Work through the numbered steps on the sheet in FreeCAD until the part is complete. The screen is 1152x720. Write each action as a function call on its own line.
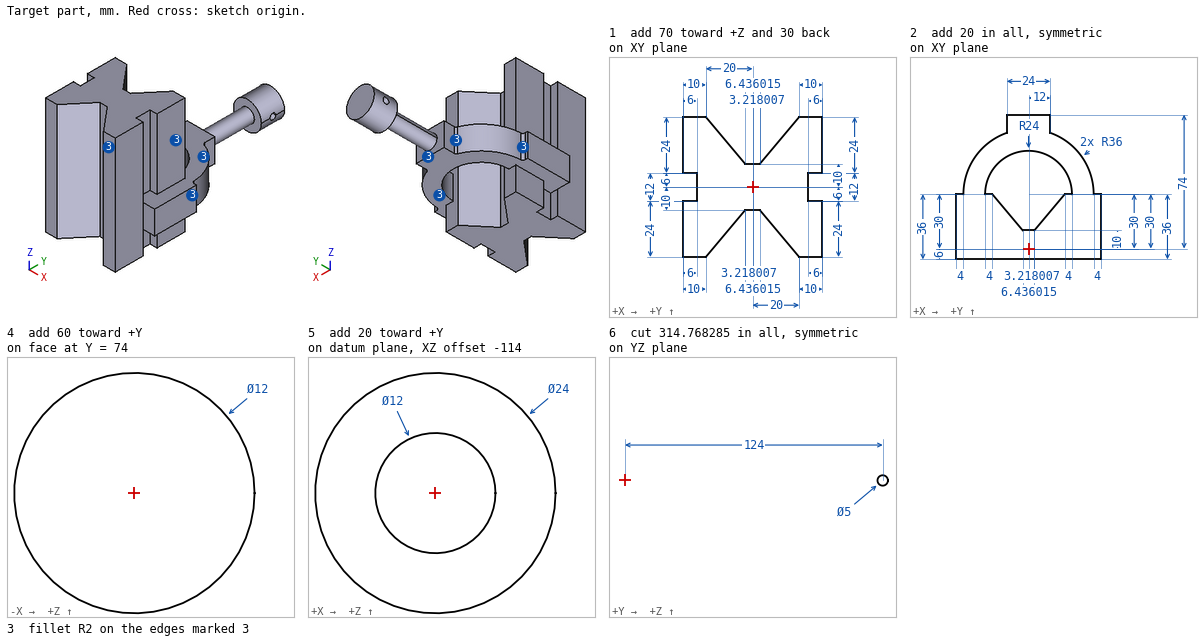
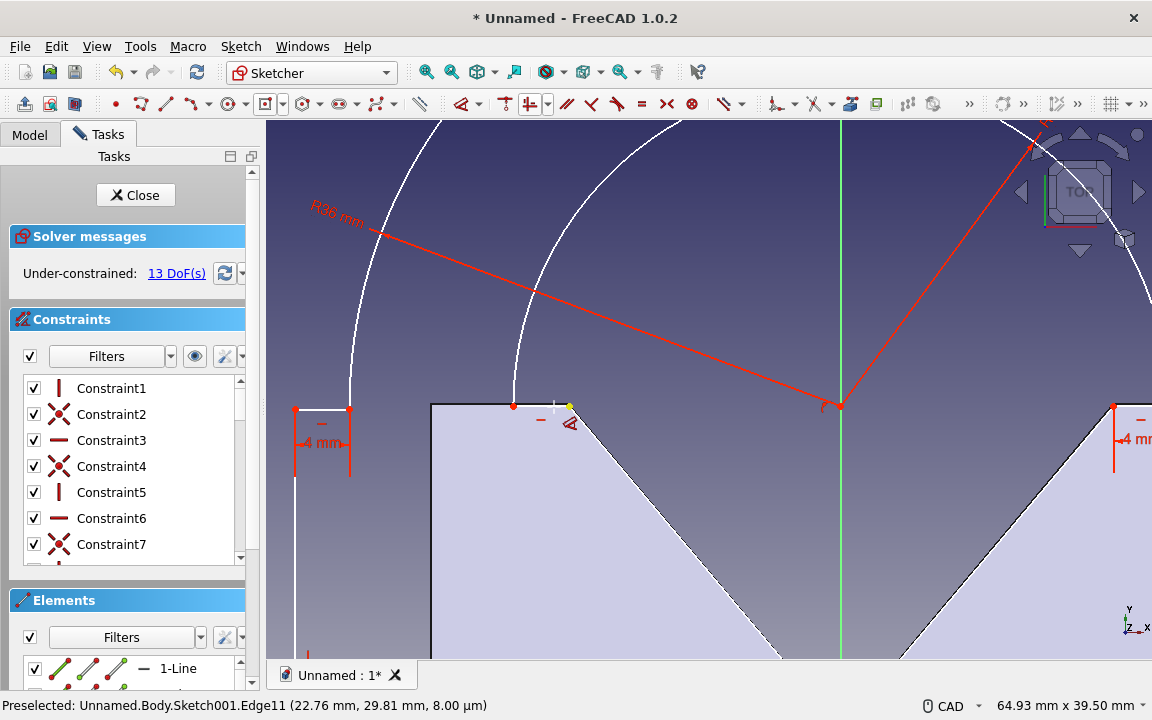
click(552, 406)
click(541, 440)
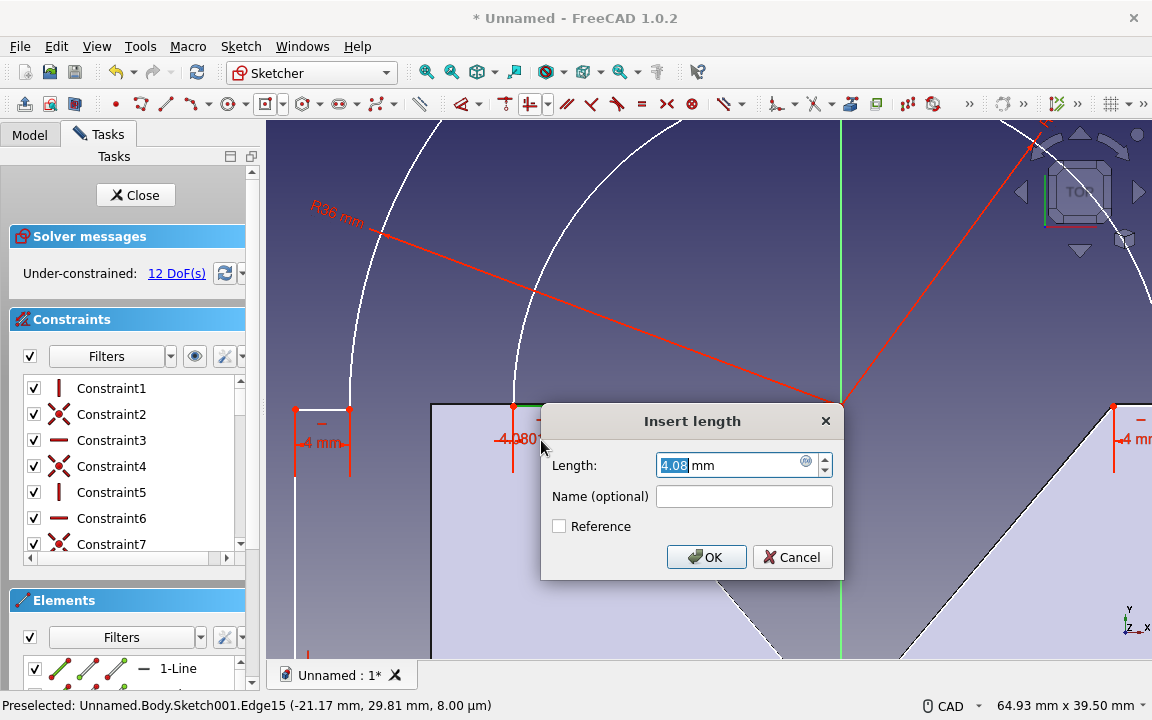
text(4)
key(Return)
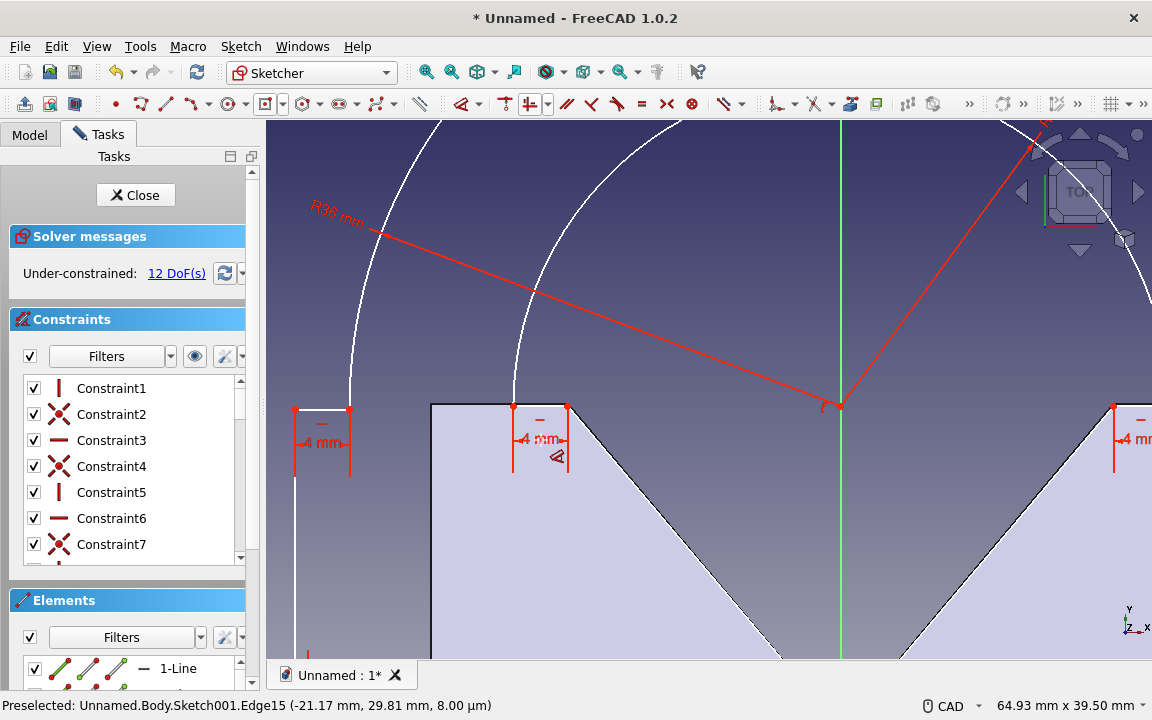
scroll(554, 407, down, 6)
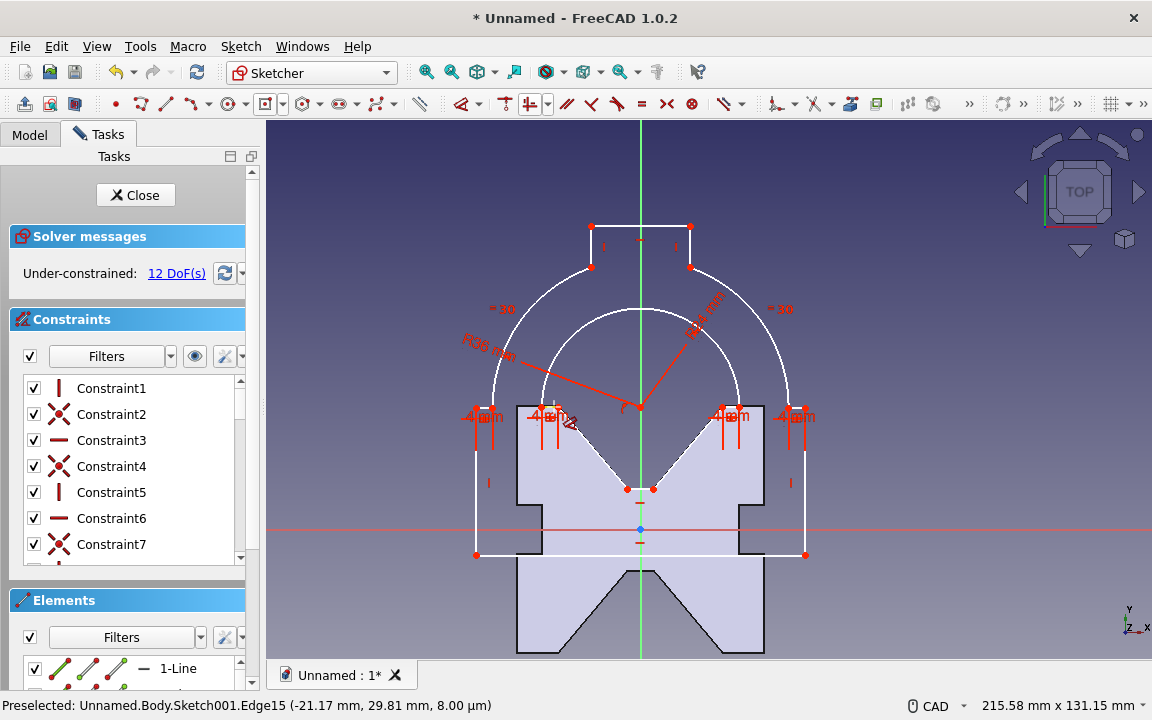
click(660, 226)
click(618, 192)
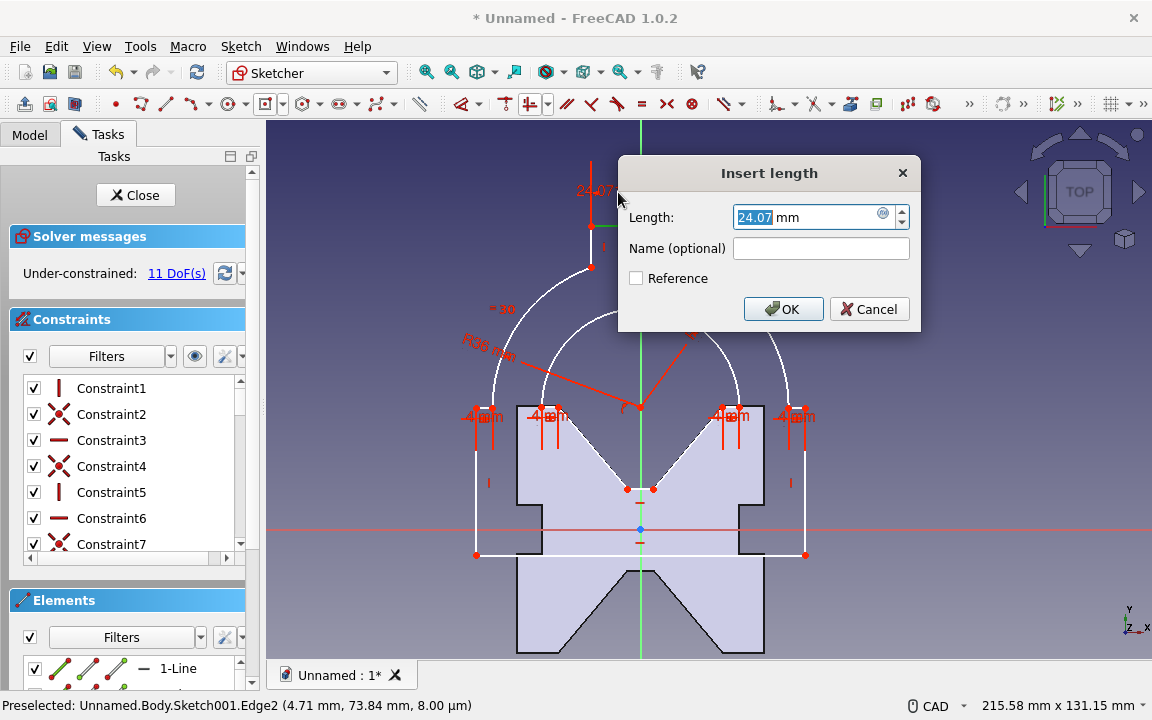
text(24)
key(Return)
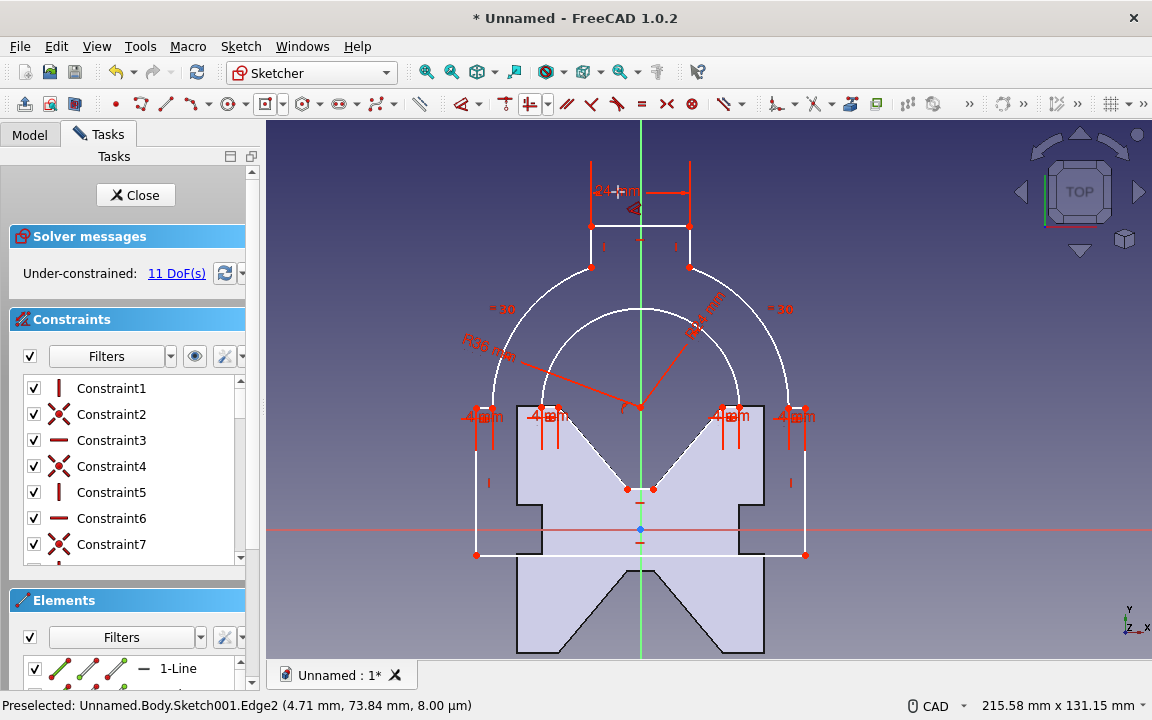
click(476, 453)
click(442, 482)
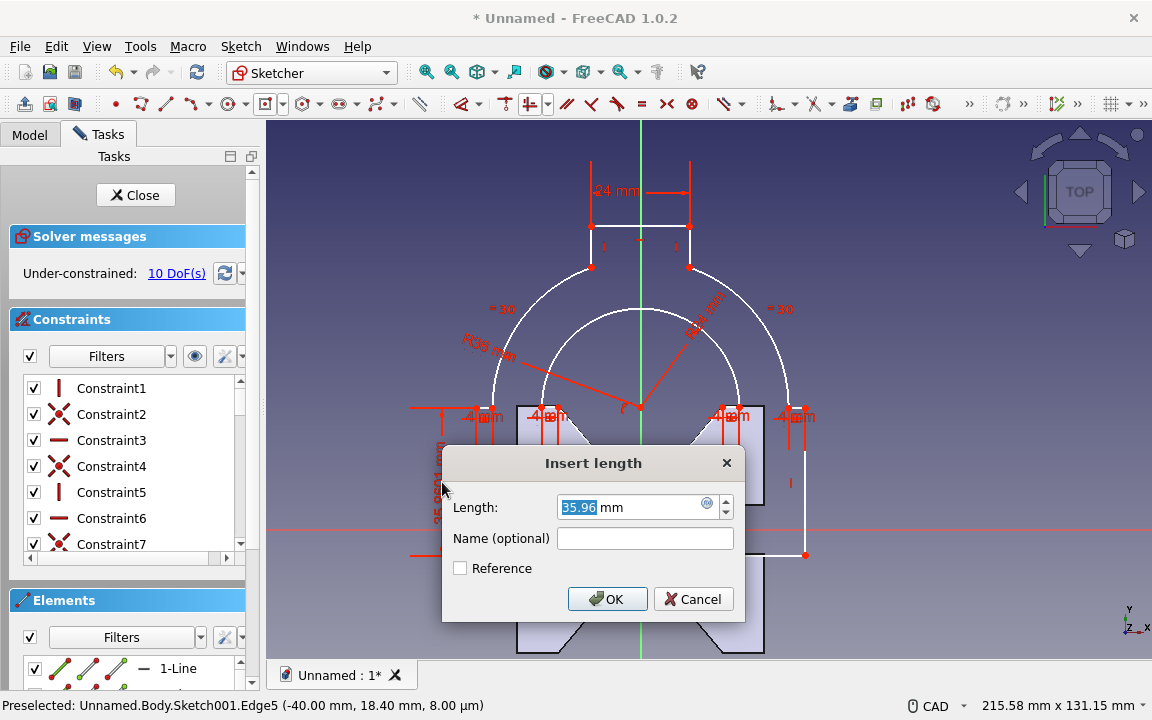
text(36)
key(Return)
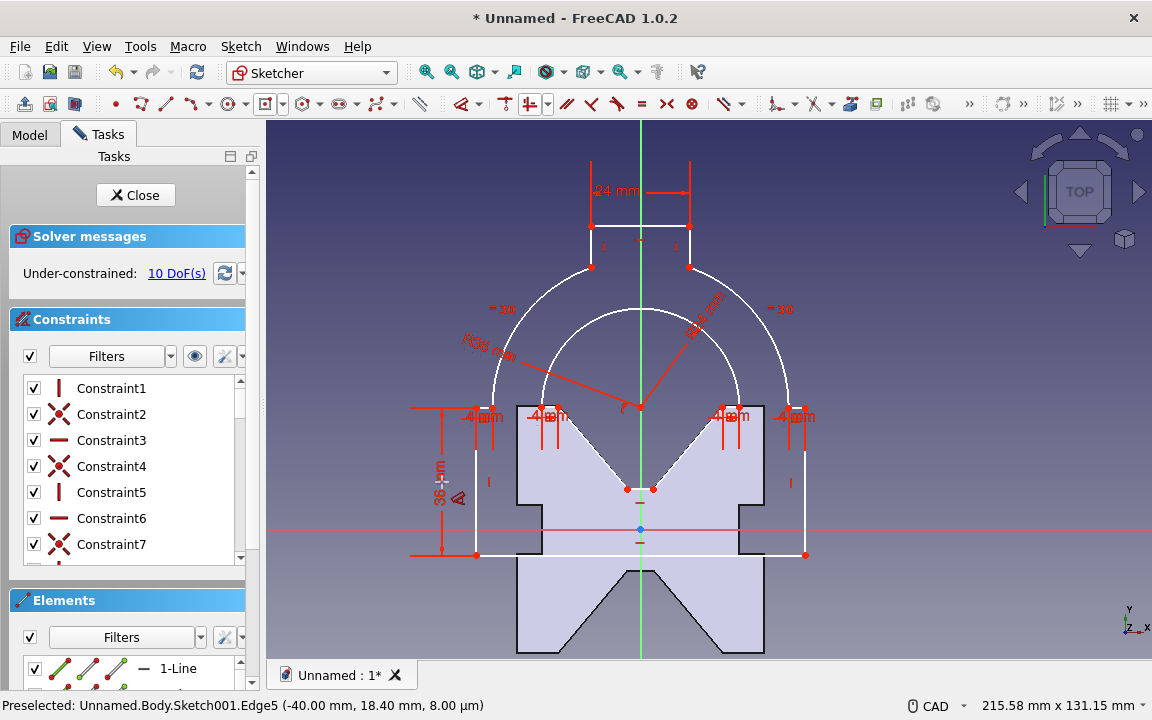
click(805, 512)
click(839, 482)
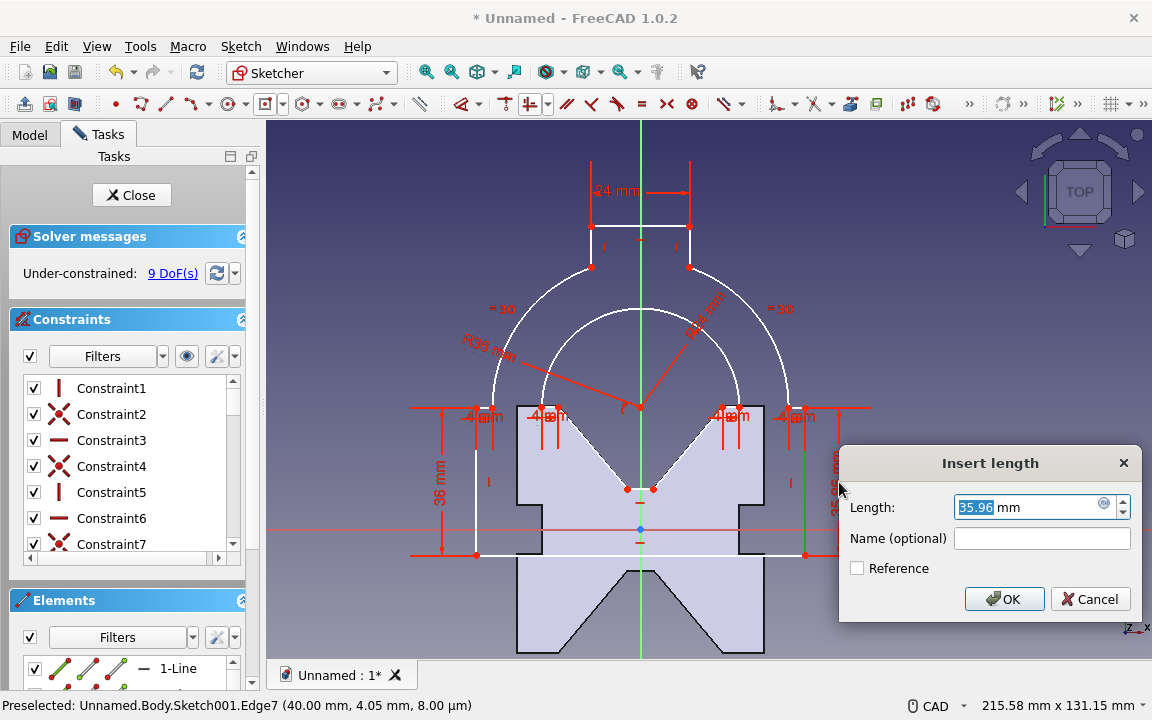
text(36)
key(Return)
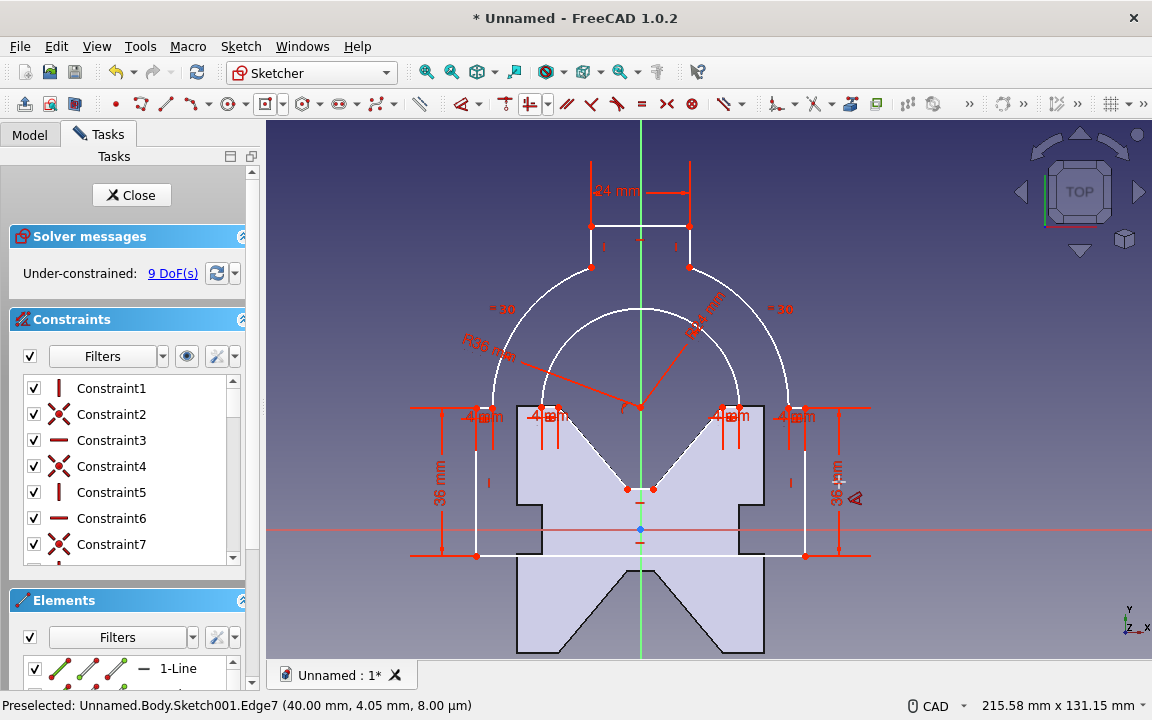
scroll(476, 556, up, 3)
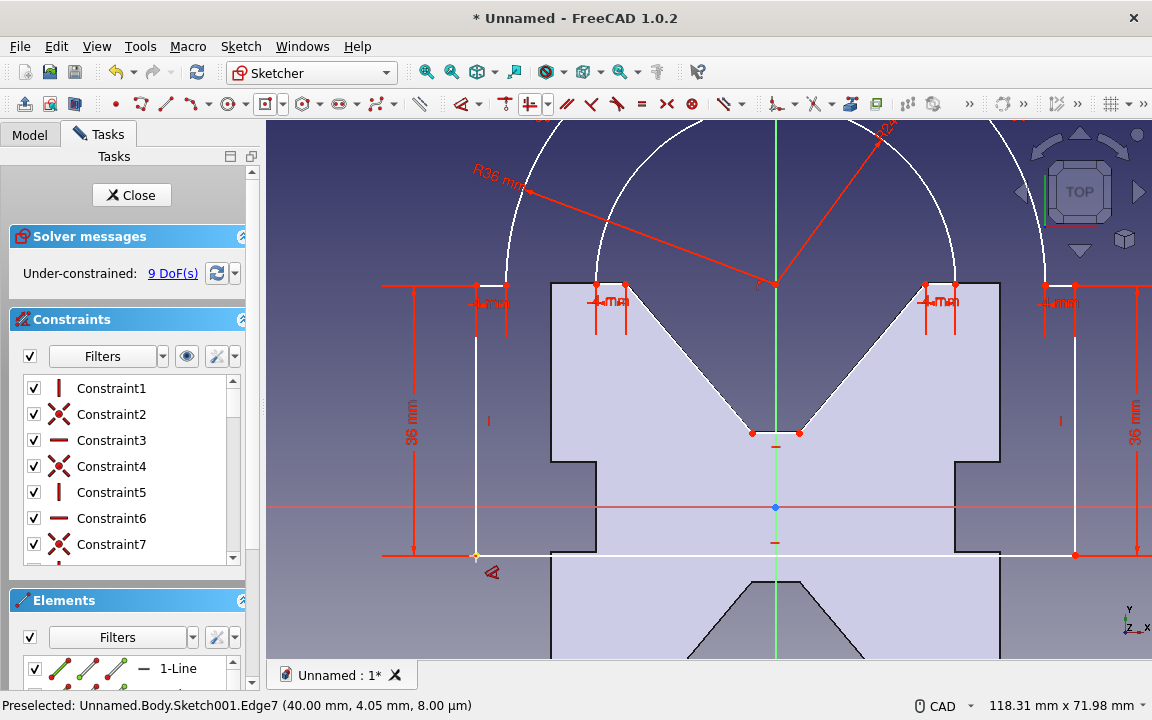
click(476, 556)
click(442, 531)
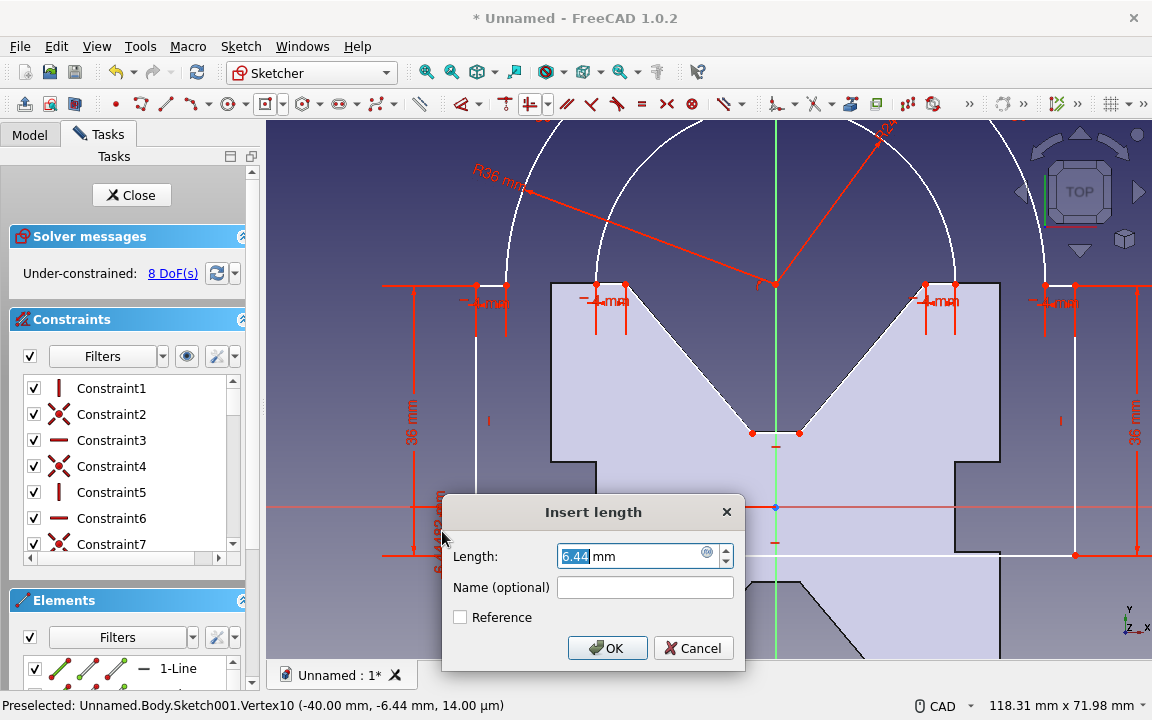
text(6)
key(Return)